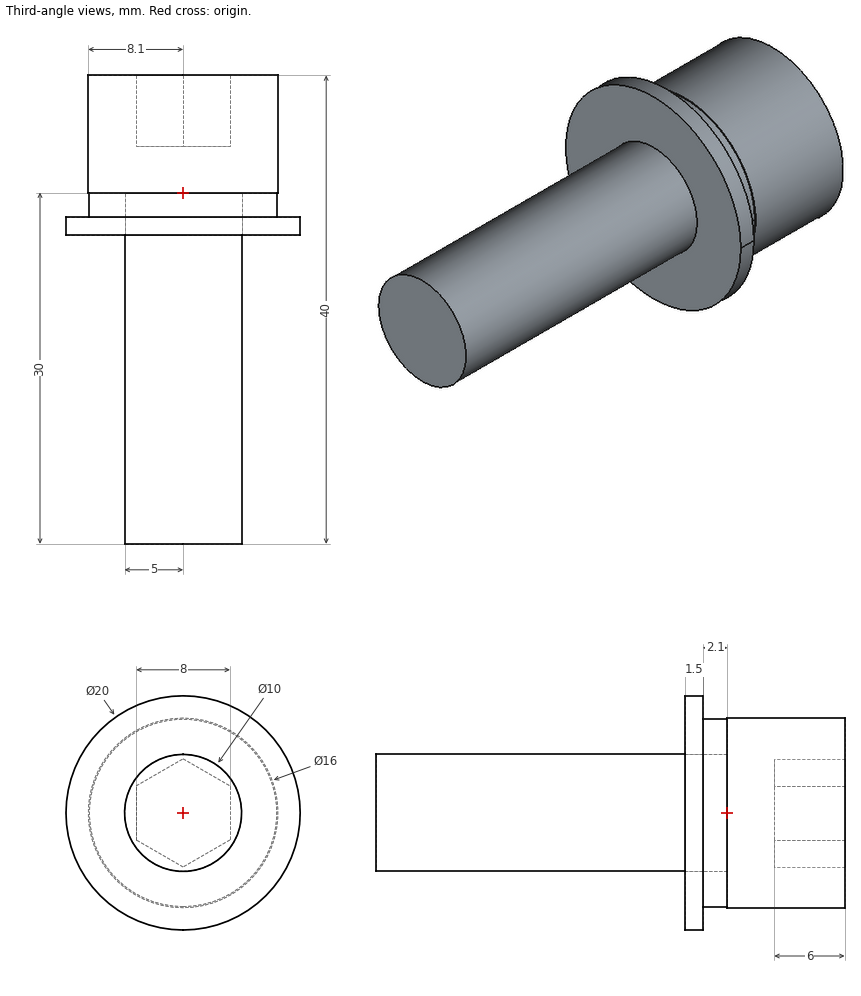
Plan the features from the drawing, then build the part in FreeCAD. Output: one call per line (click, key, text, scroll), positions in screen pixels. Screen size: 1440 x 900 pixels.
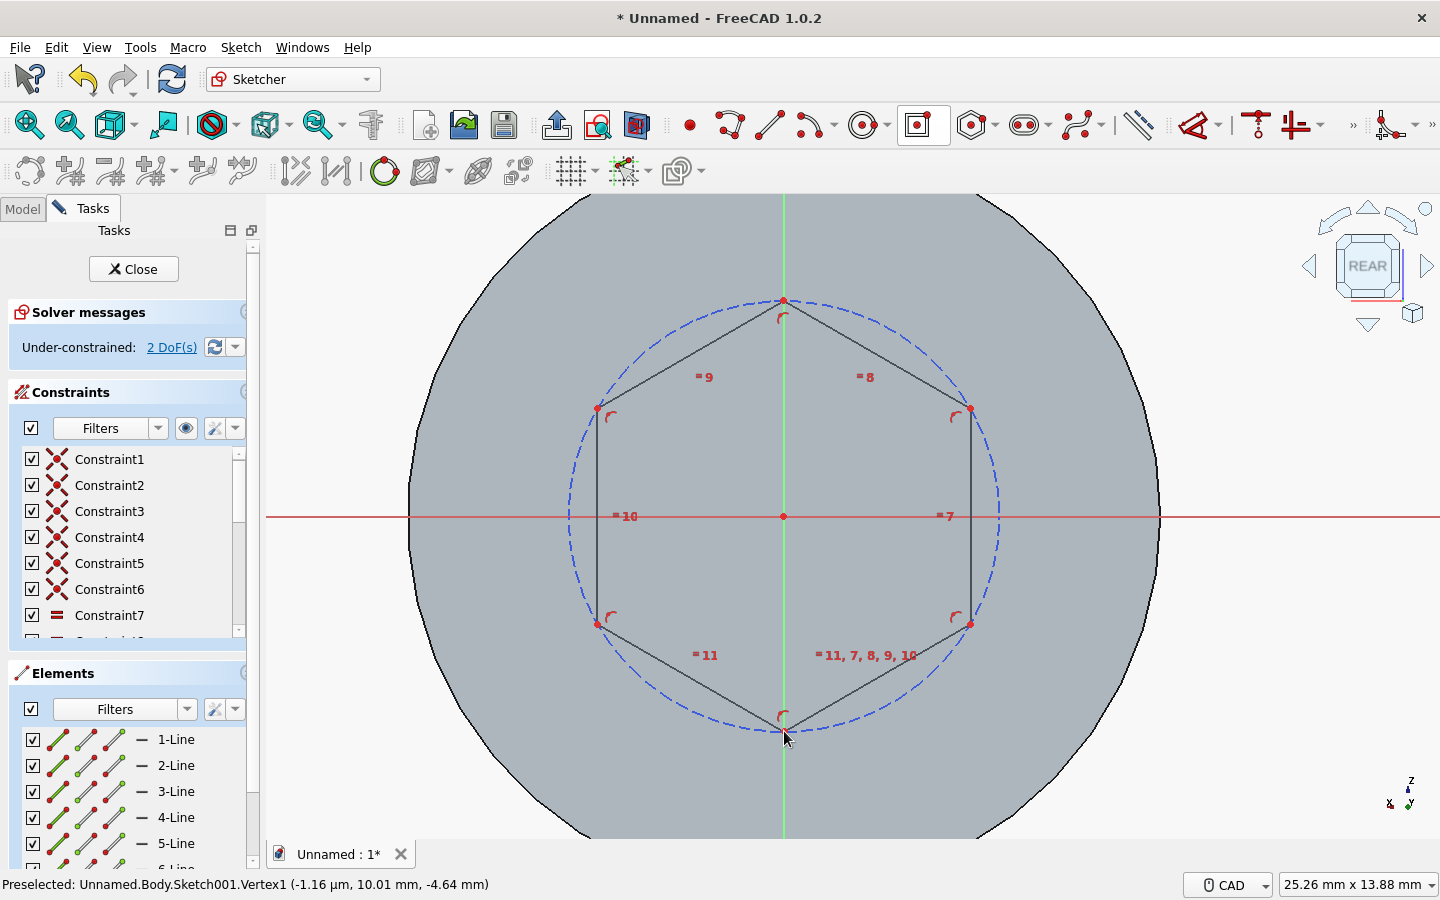
click(971, 560)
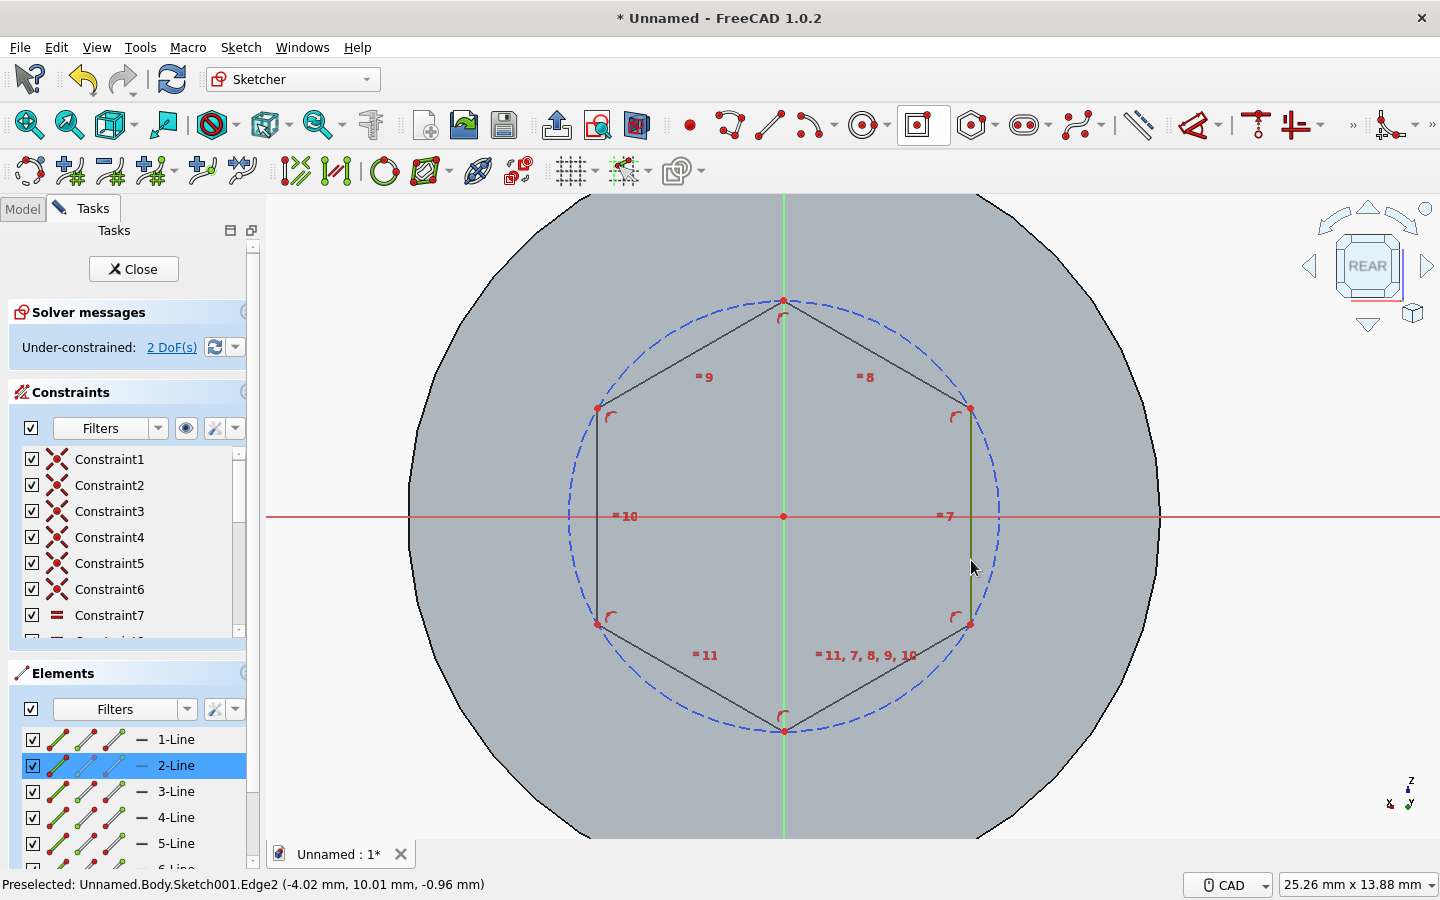
click(1322, 126)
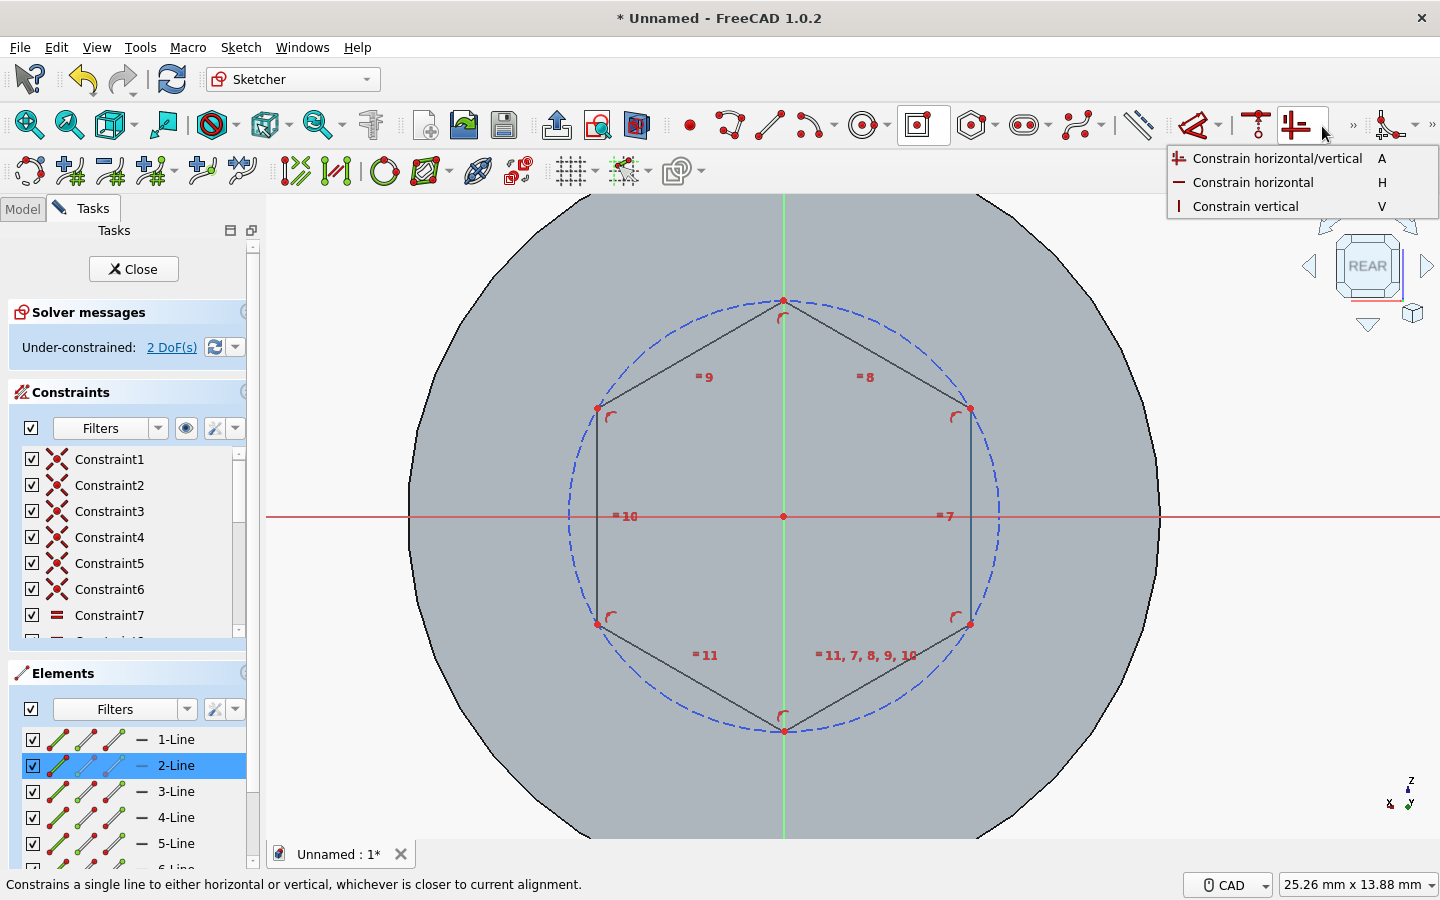
click(1303, 206)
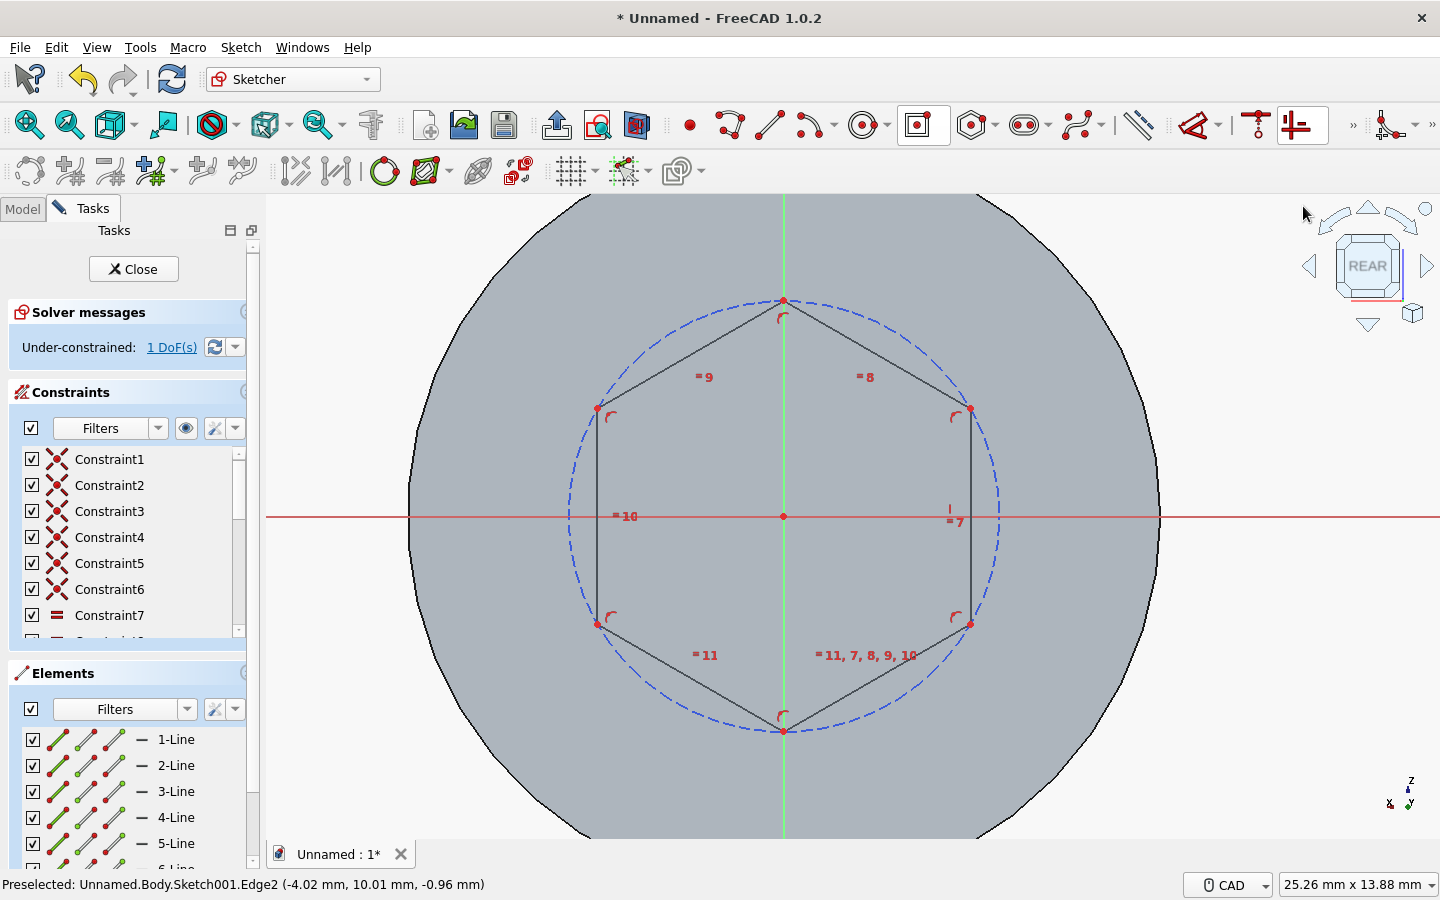
click(1194, 126)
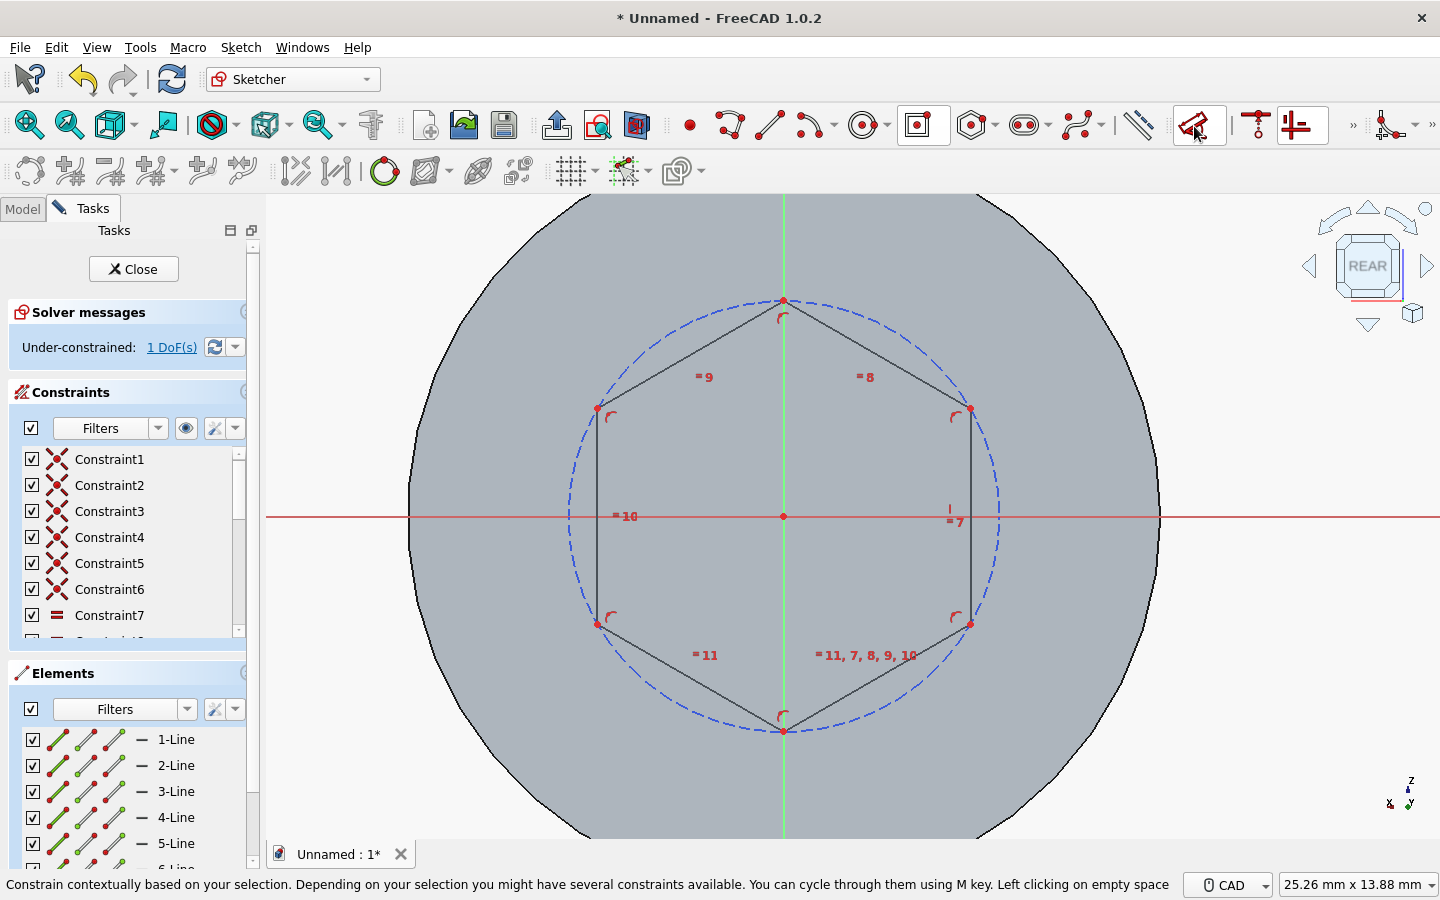
click(597, 409)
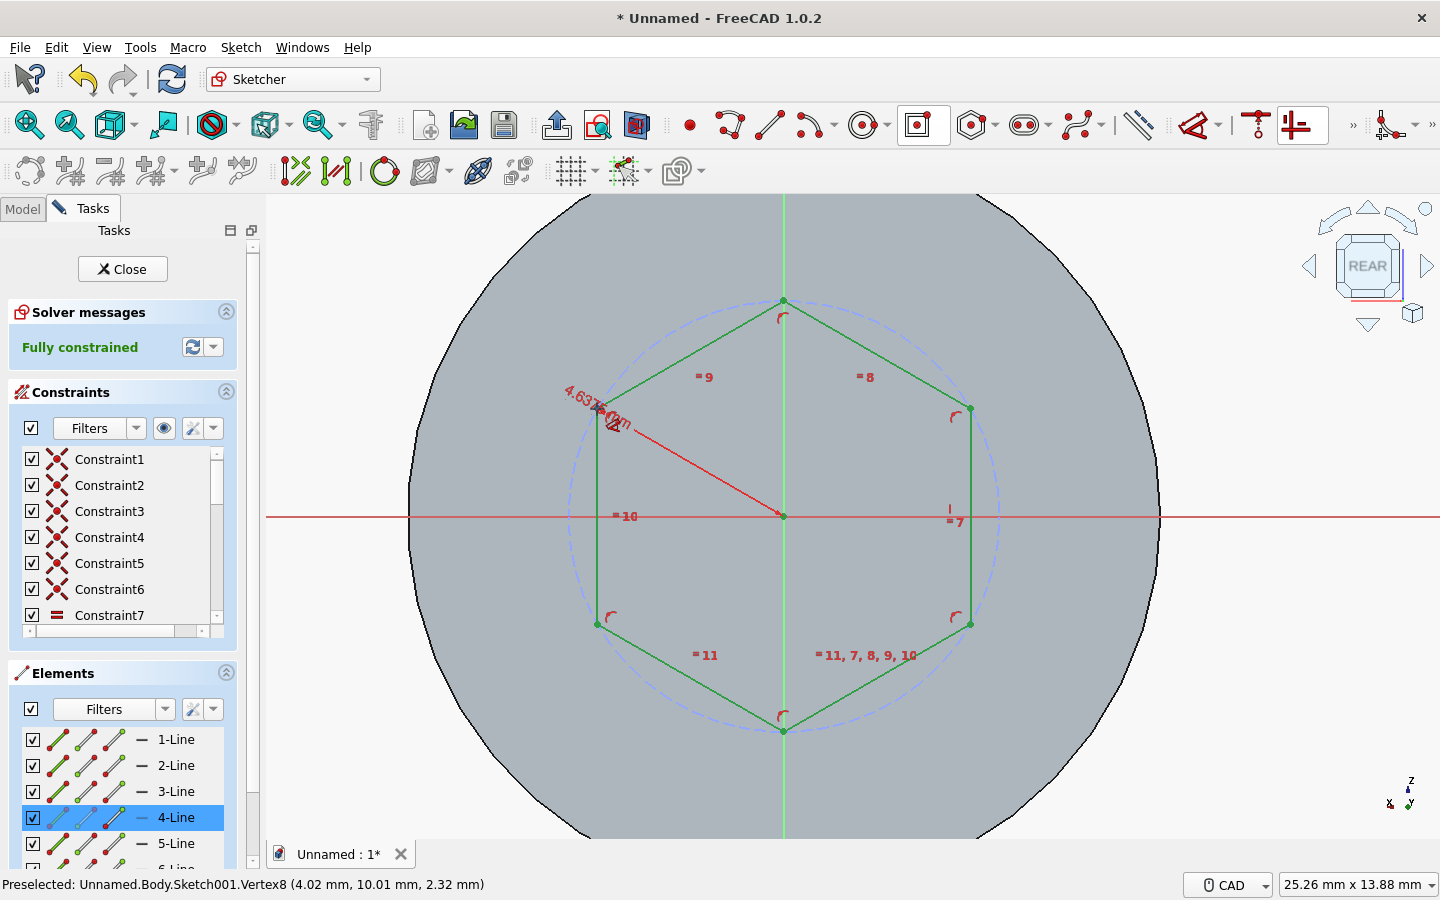
click(971, 624)
click(698, 658)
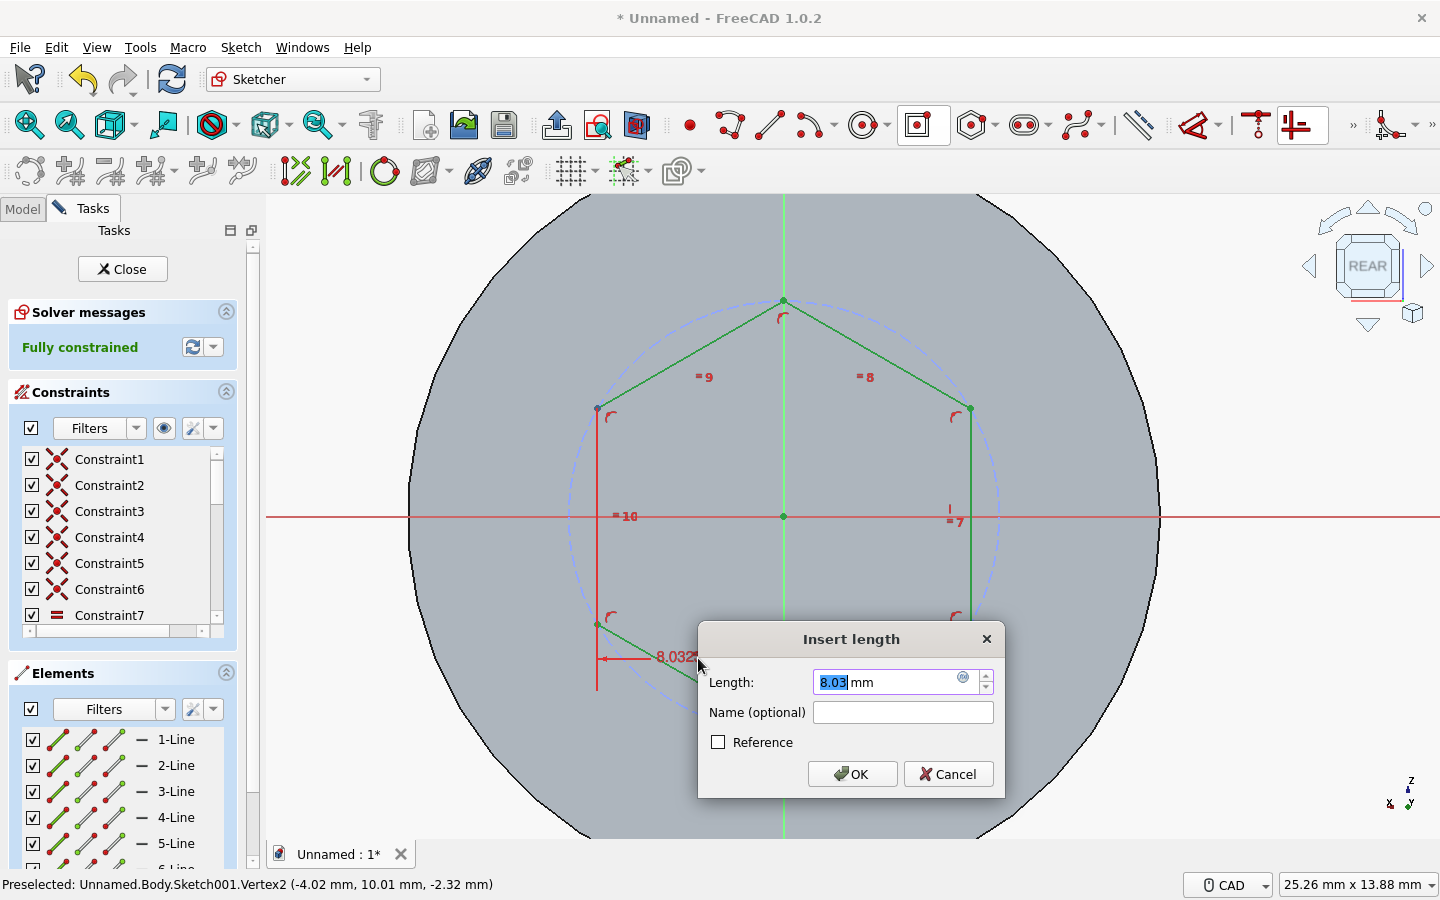
text(8)
key(Return)
key(Escape)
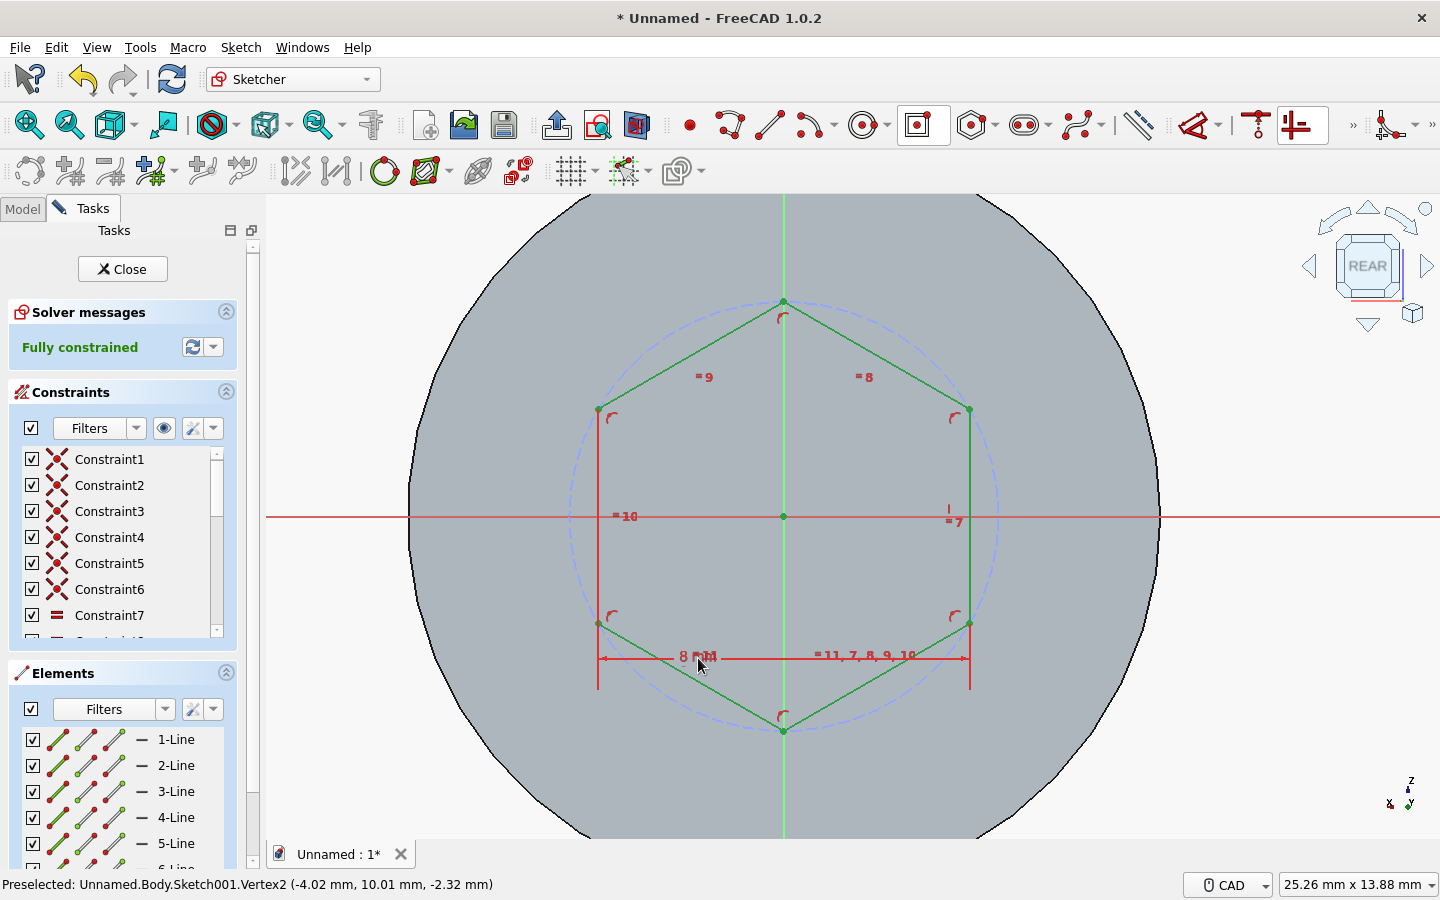
click(123, 269)